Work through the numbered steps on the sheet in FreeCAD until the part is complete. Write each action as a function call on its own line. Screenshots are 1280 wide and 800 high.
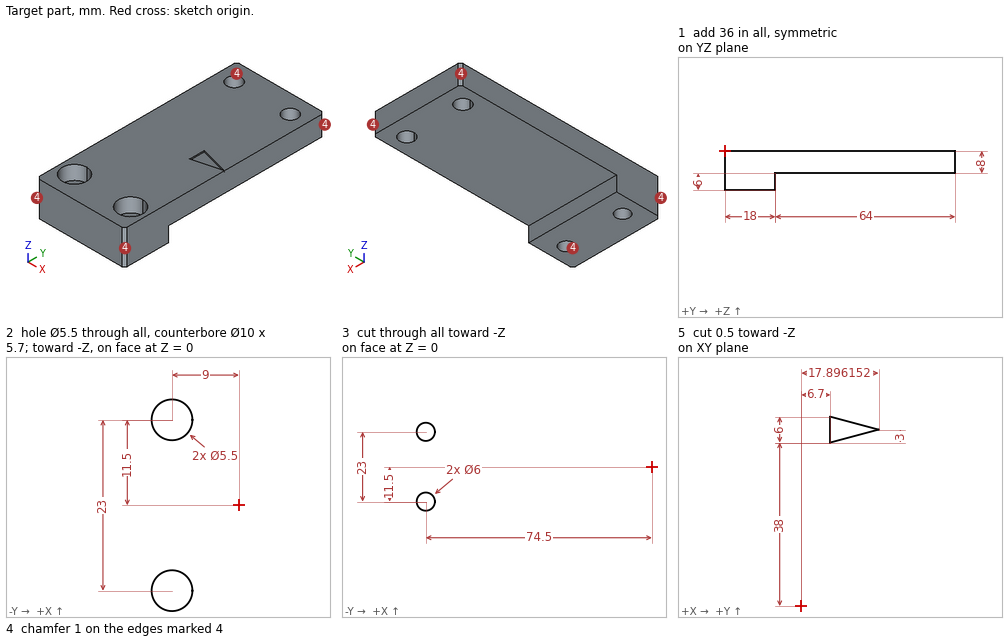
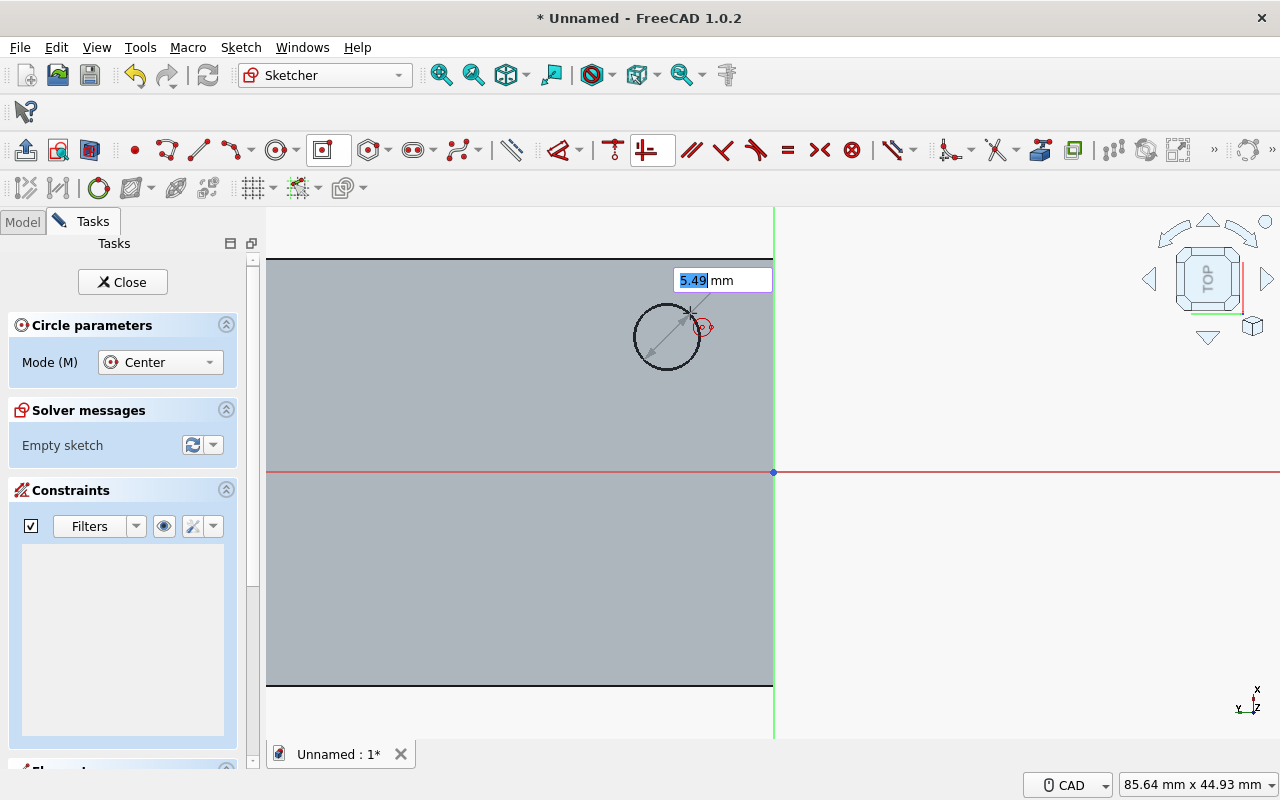
text(5.5)
key(Return)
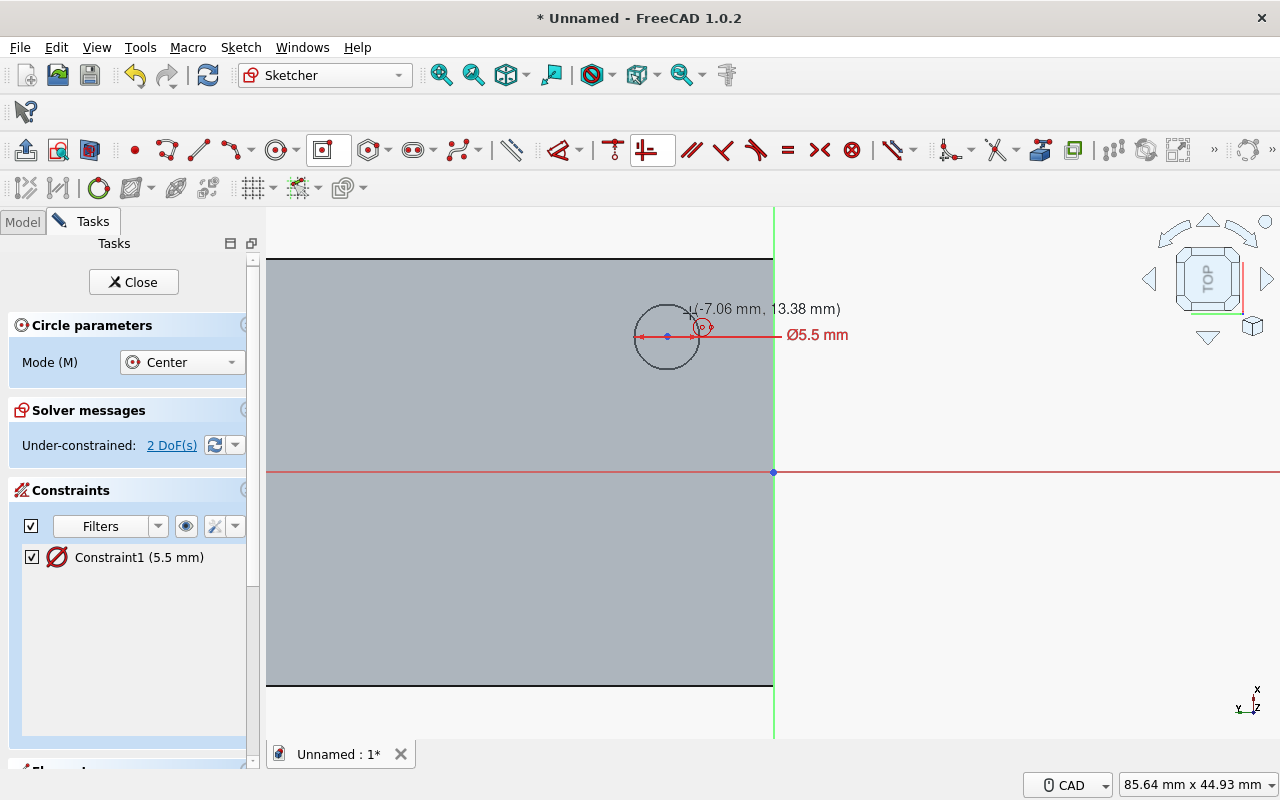
click(667, 609)
move(690, 586)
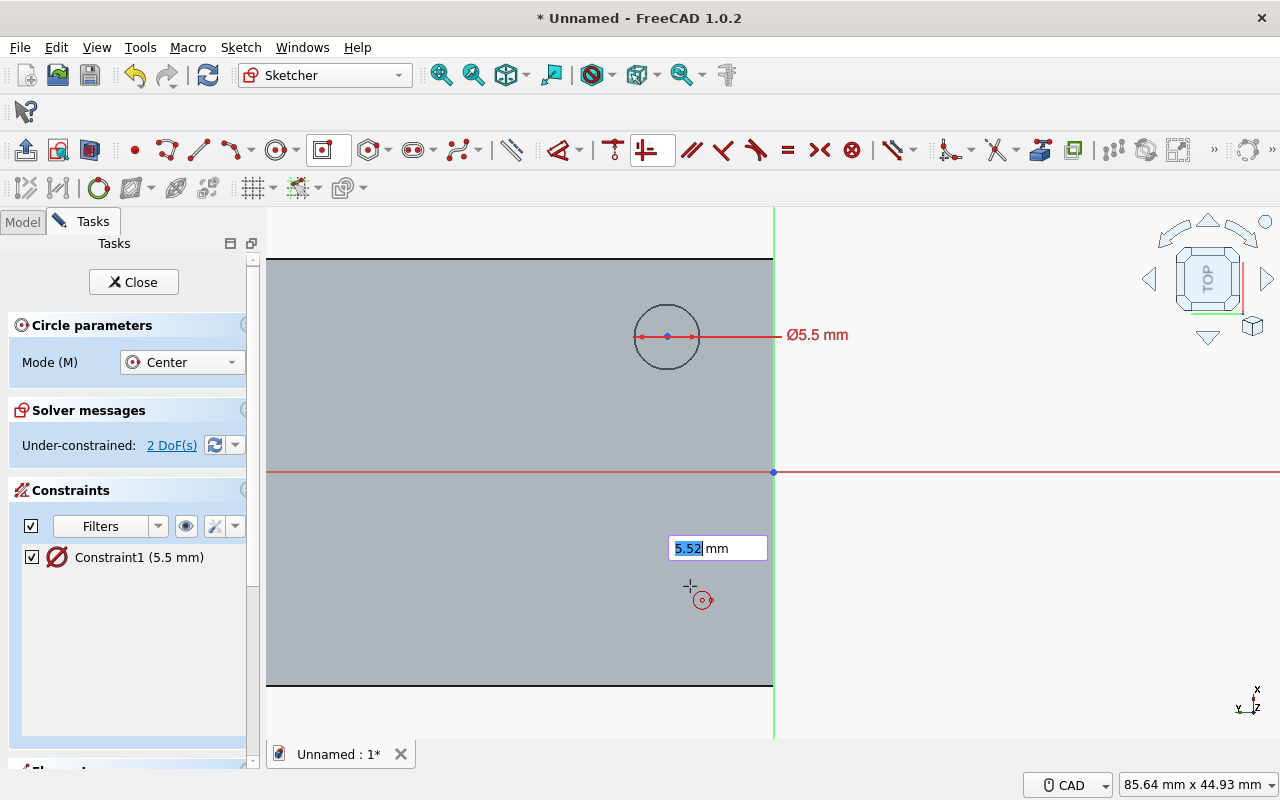
text(5.5)
key(Return)
key(Escape)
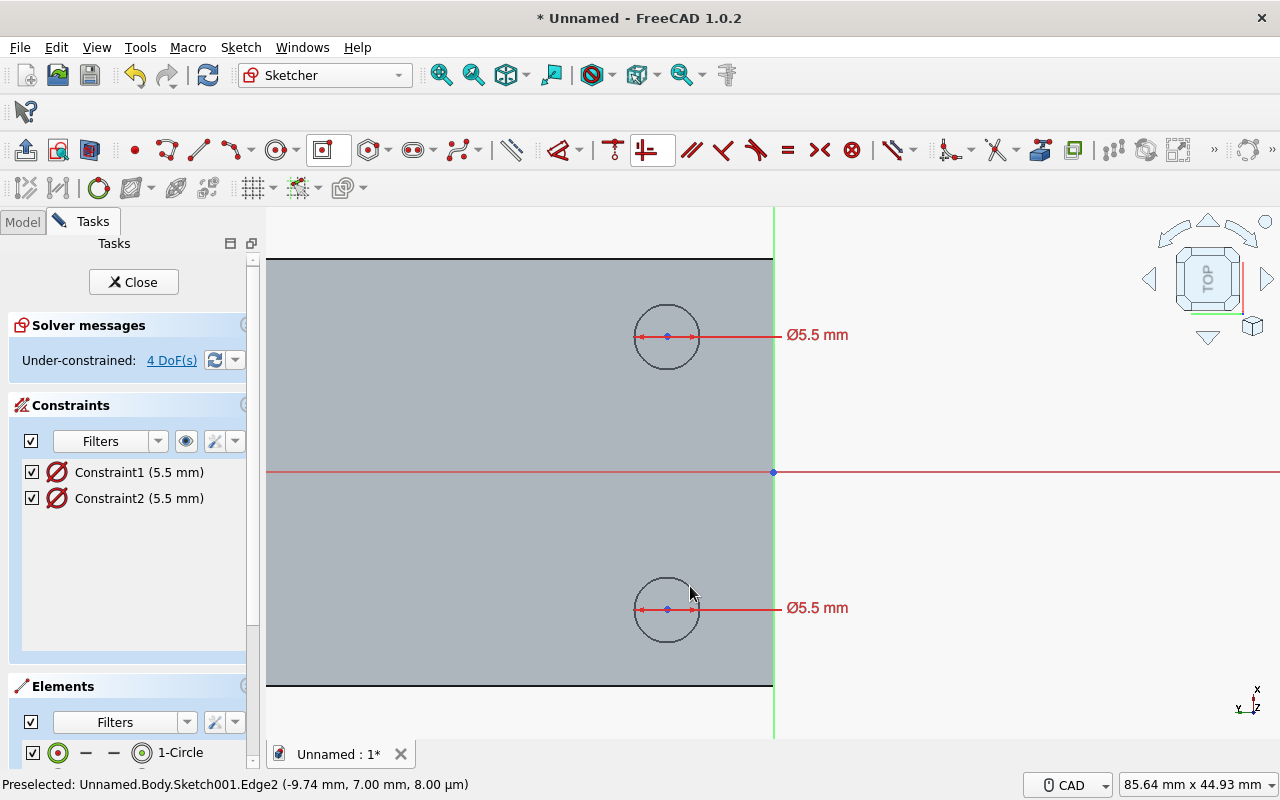
click(667, 337)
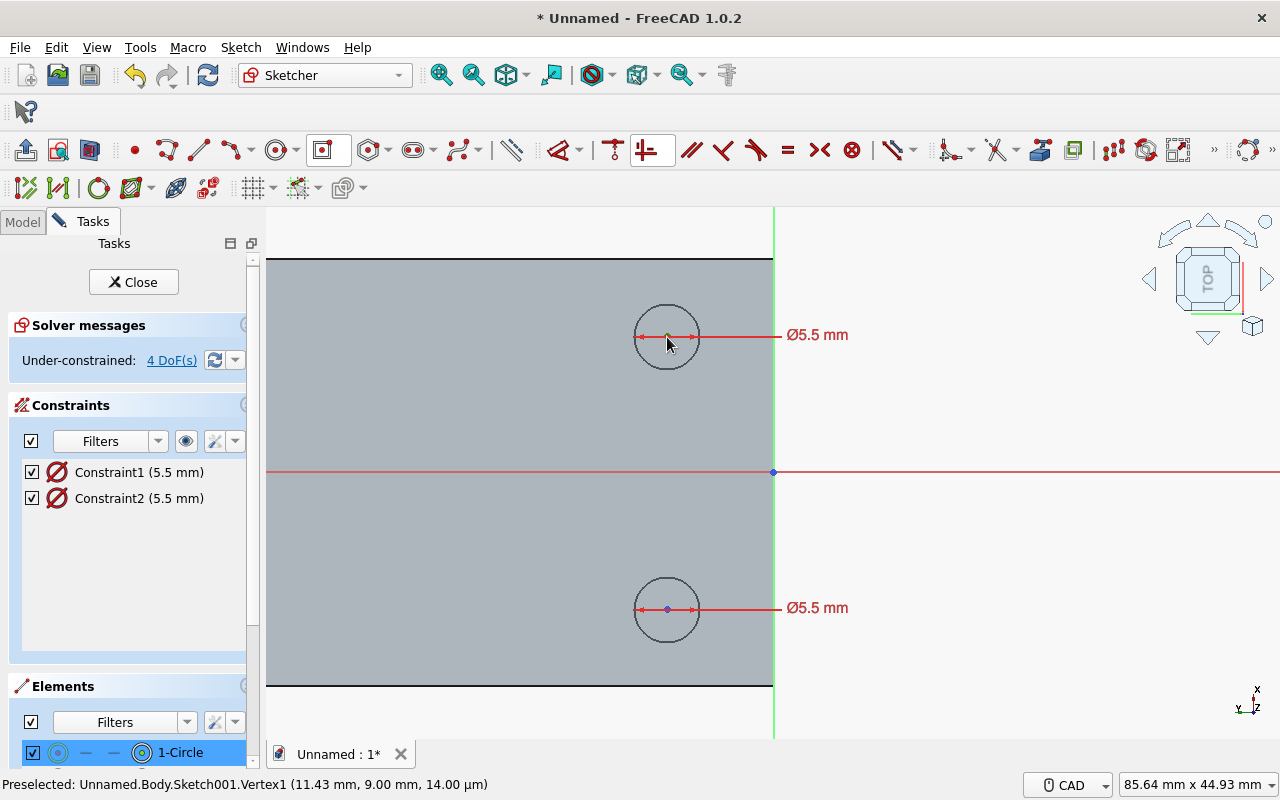
click(667, 610)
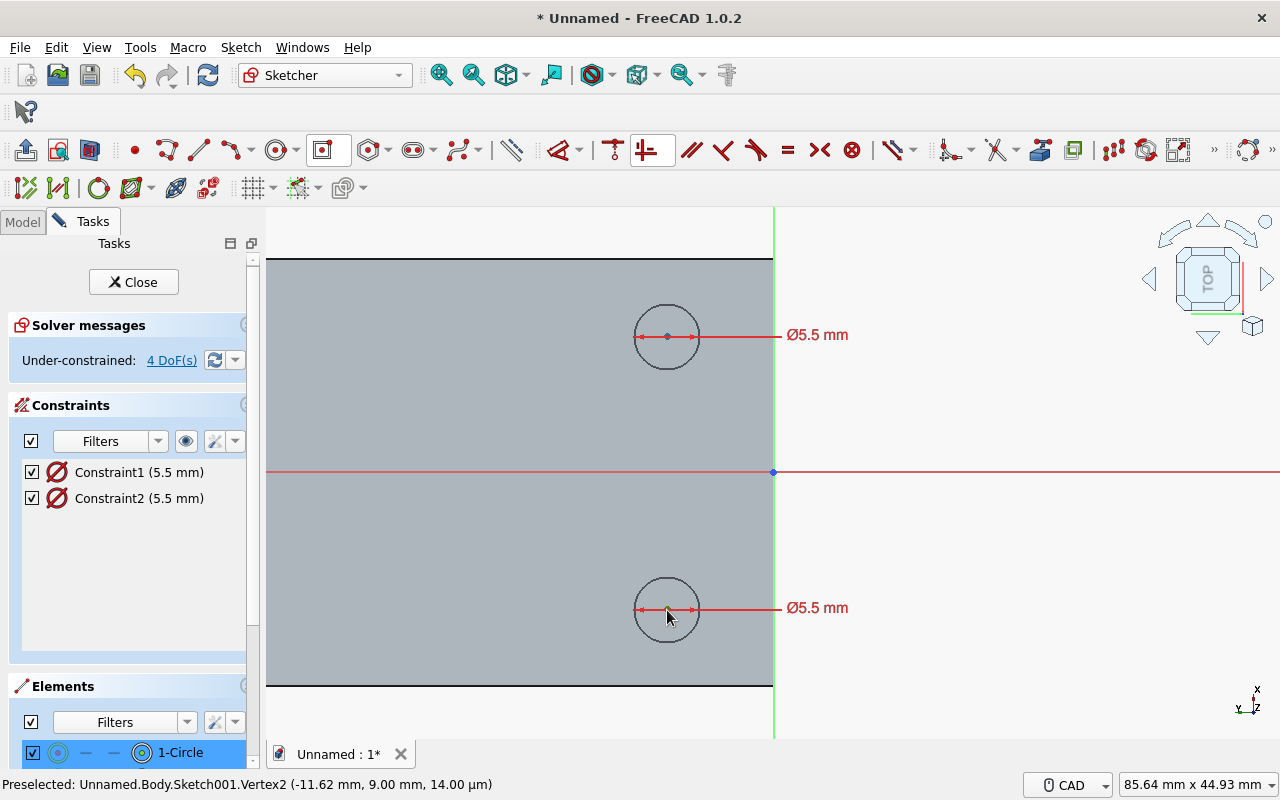
key(v)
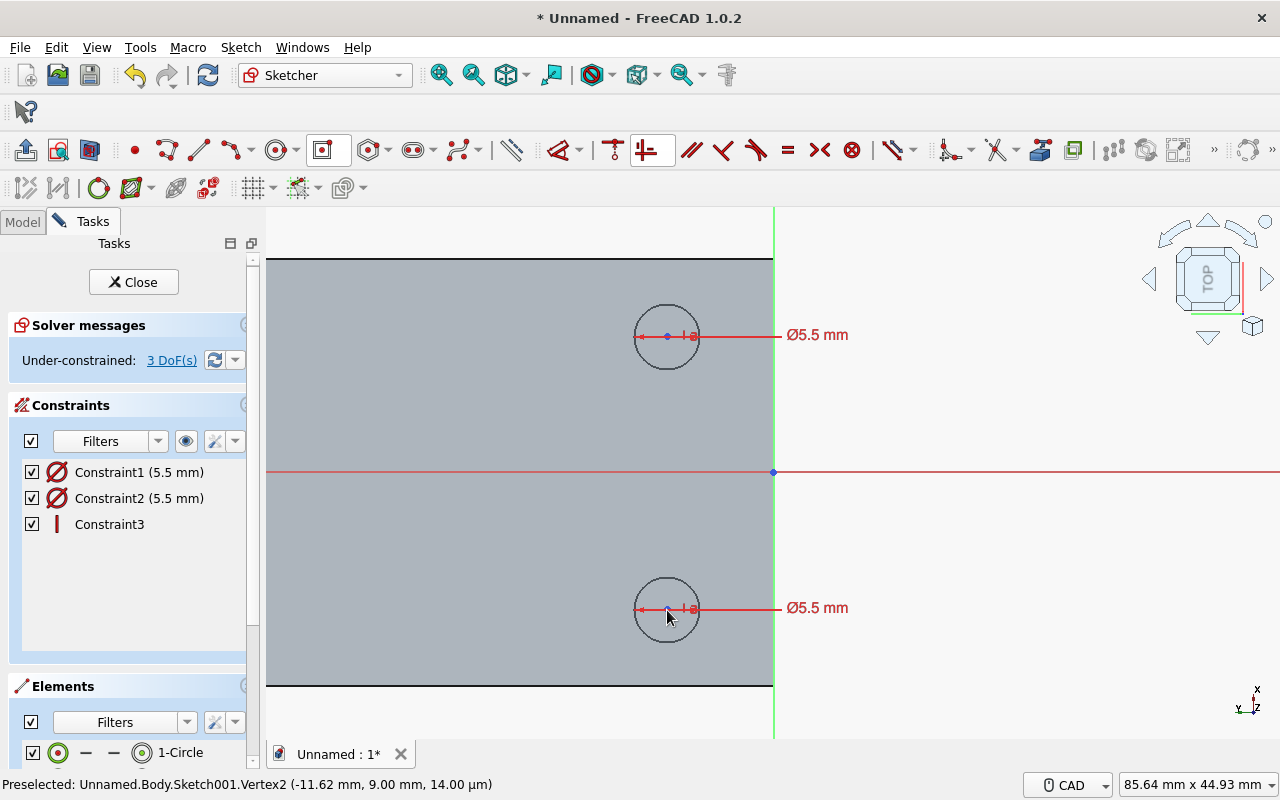
click(558, 150)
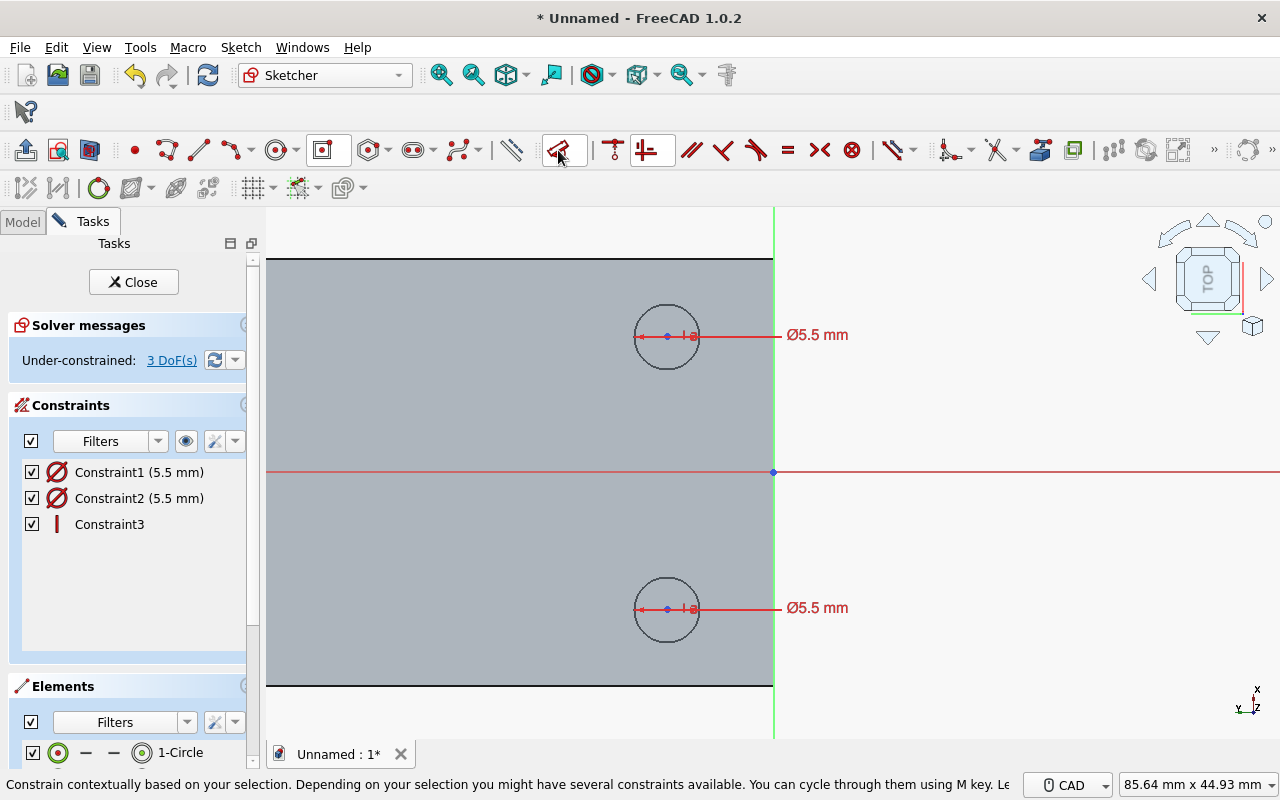
click(667, 337)
click(720, 303)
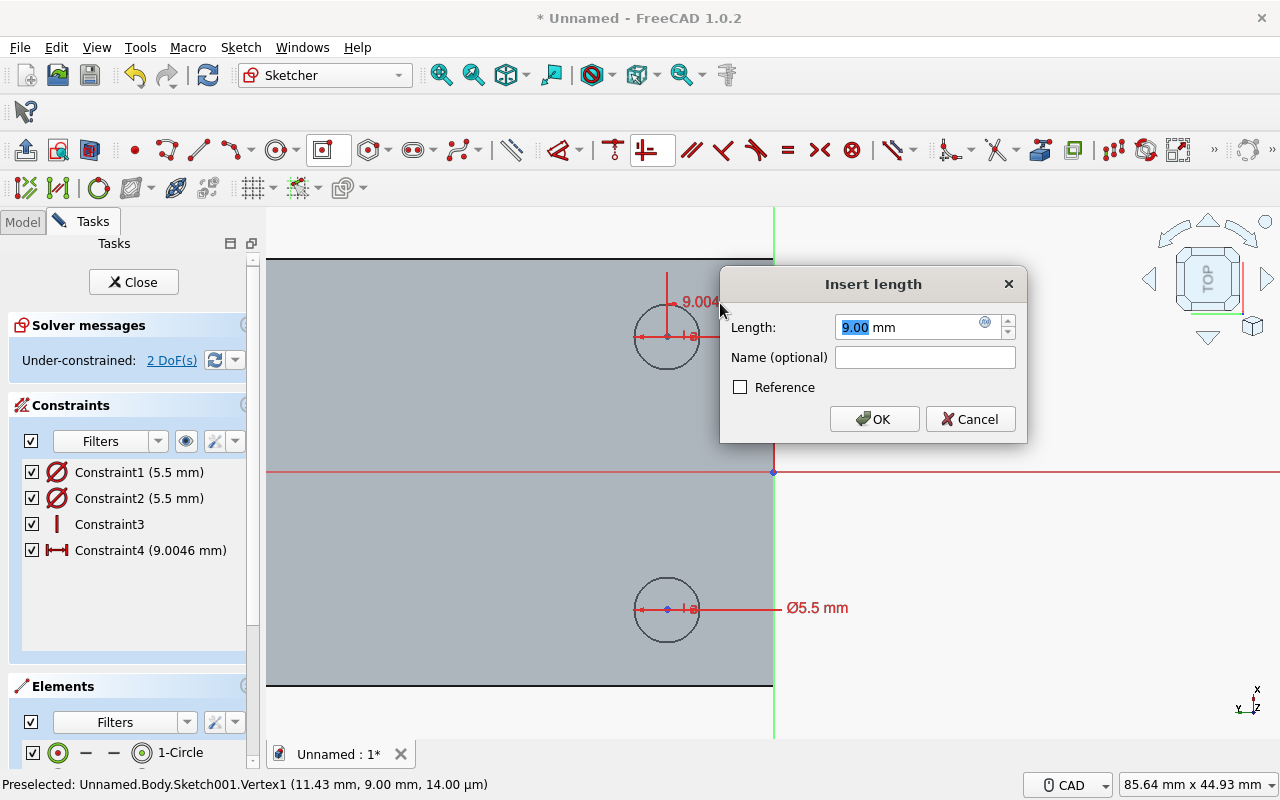
text(9)
key(Return)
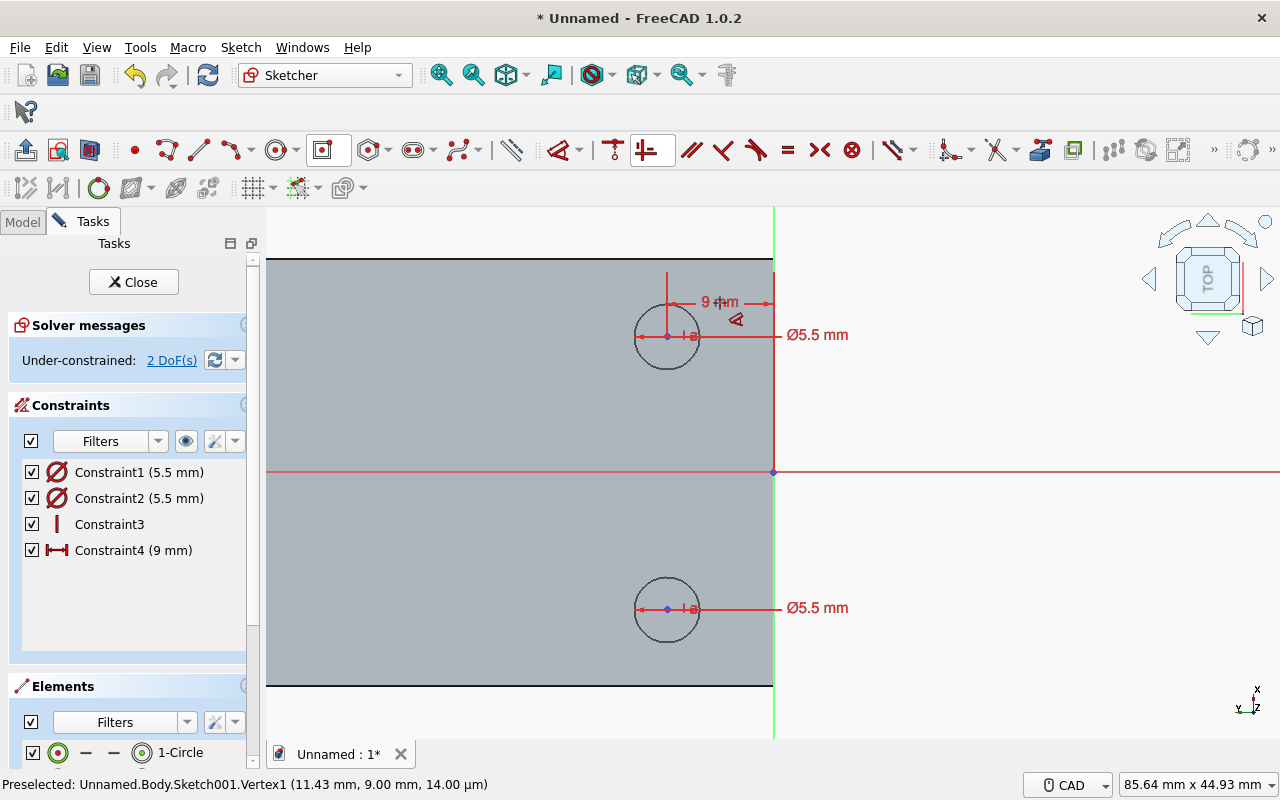
click(667, 337)